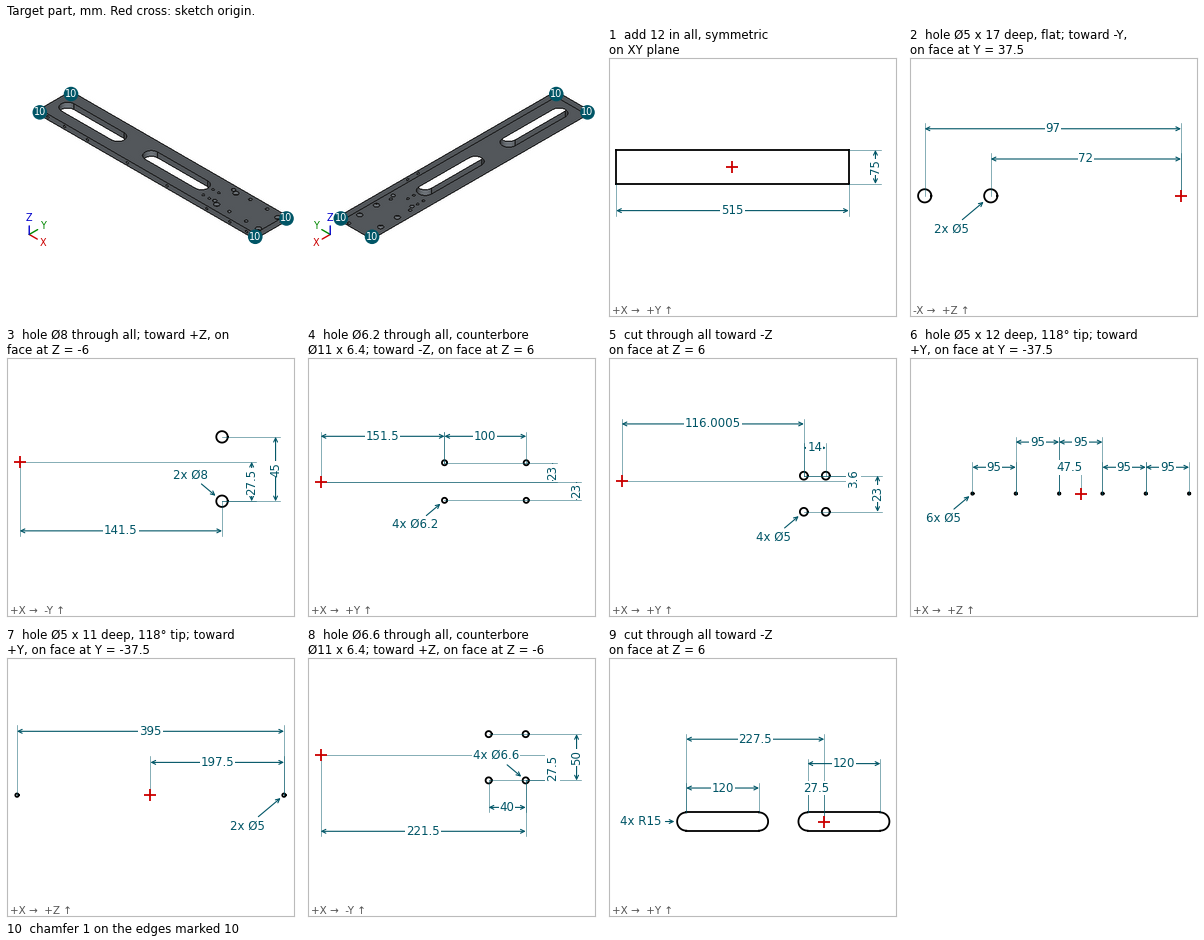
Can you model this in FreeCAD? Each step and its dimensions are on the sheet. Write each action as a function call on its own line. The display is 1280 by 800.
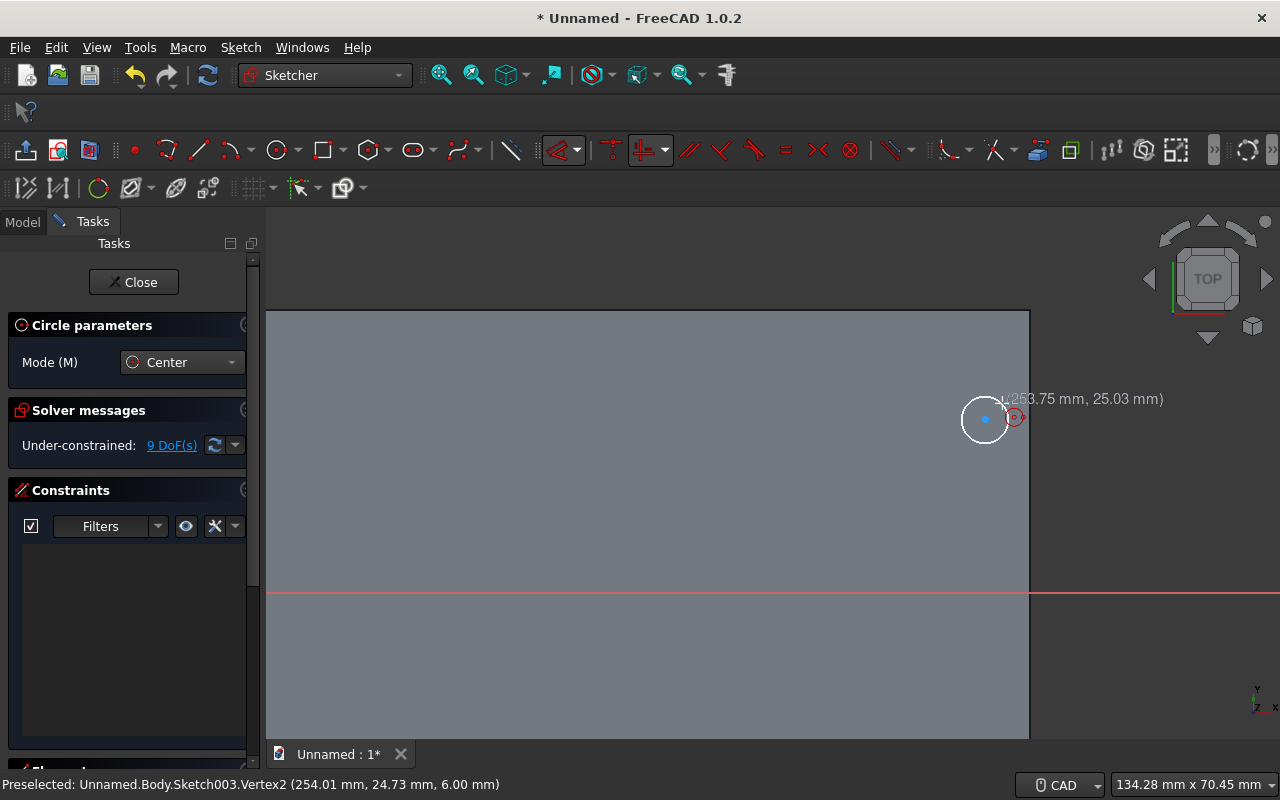
scroll(988, 421, down, 6)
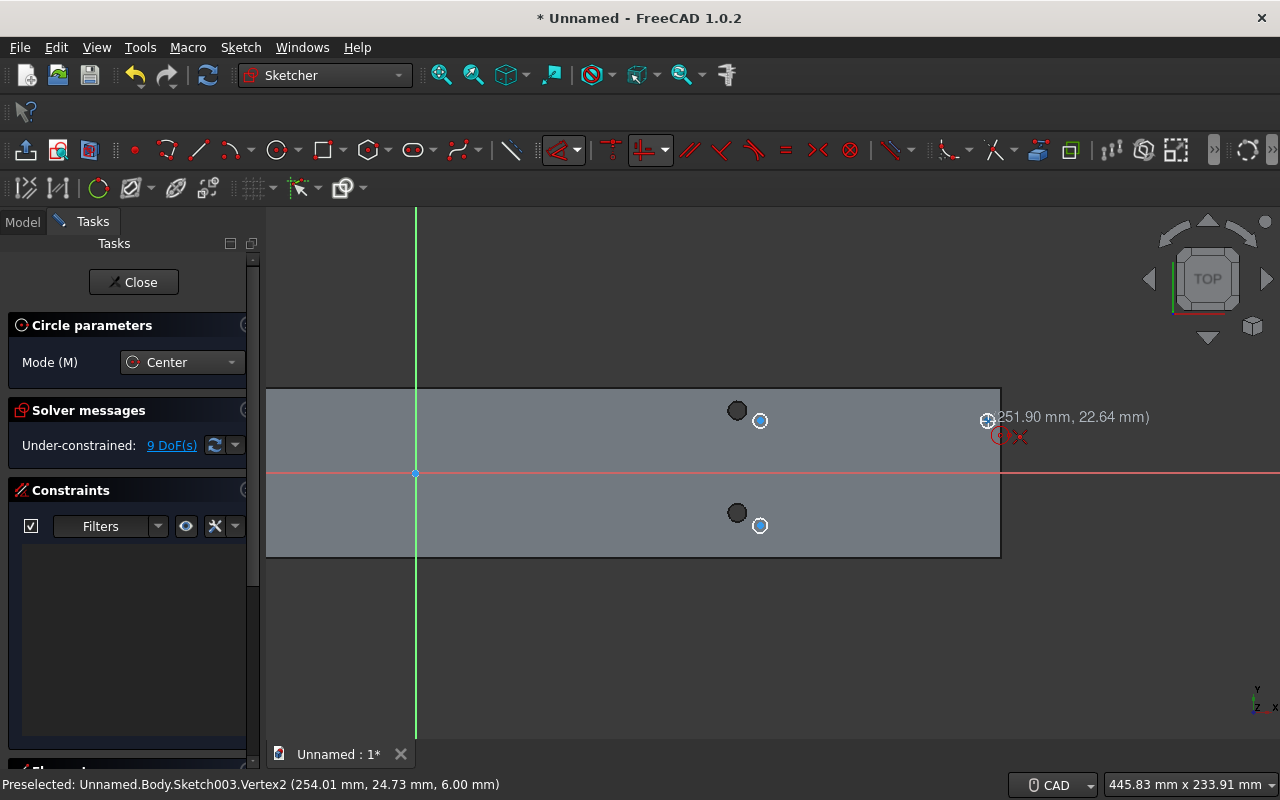
scroll(988, 525, up, 6)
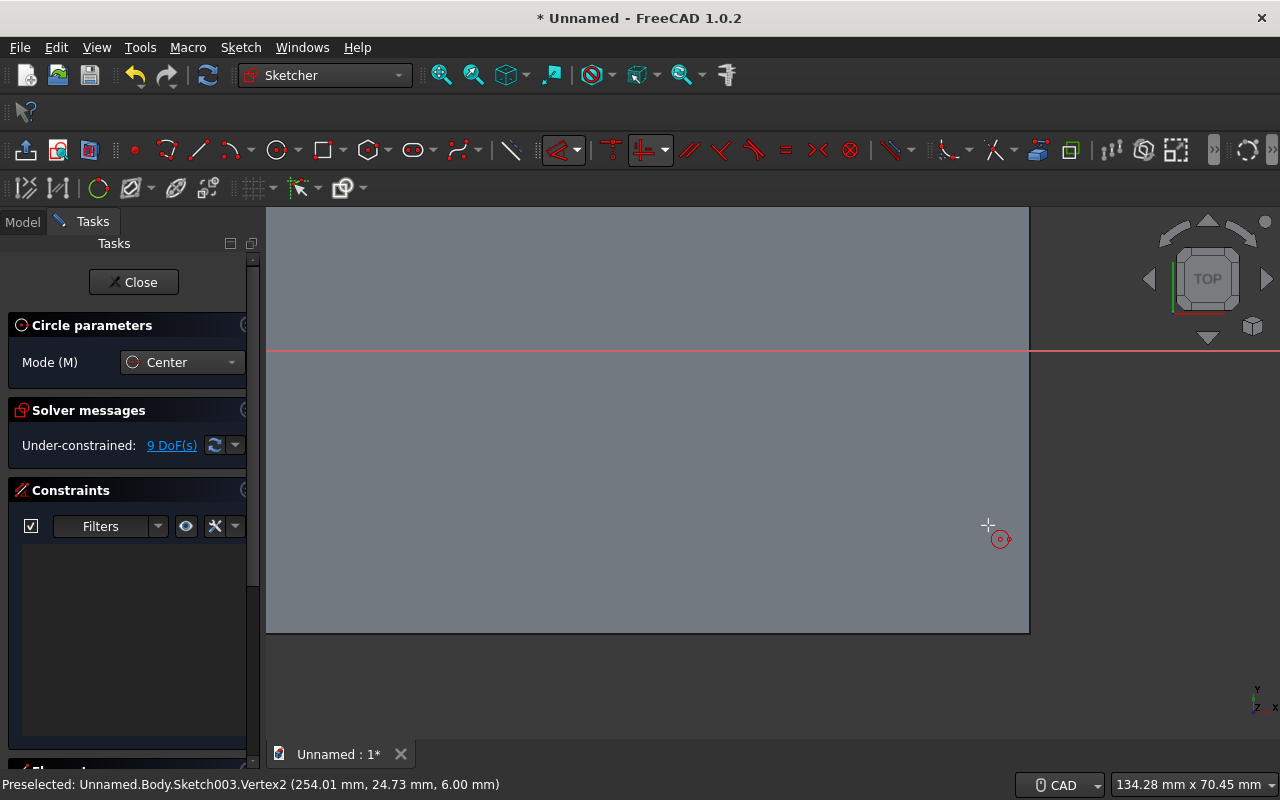
click(985, 525)
click(1002, 508)
key(Escape)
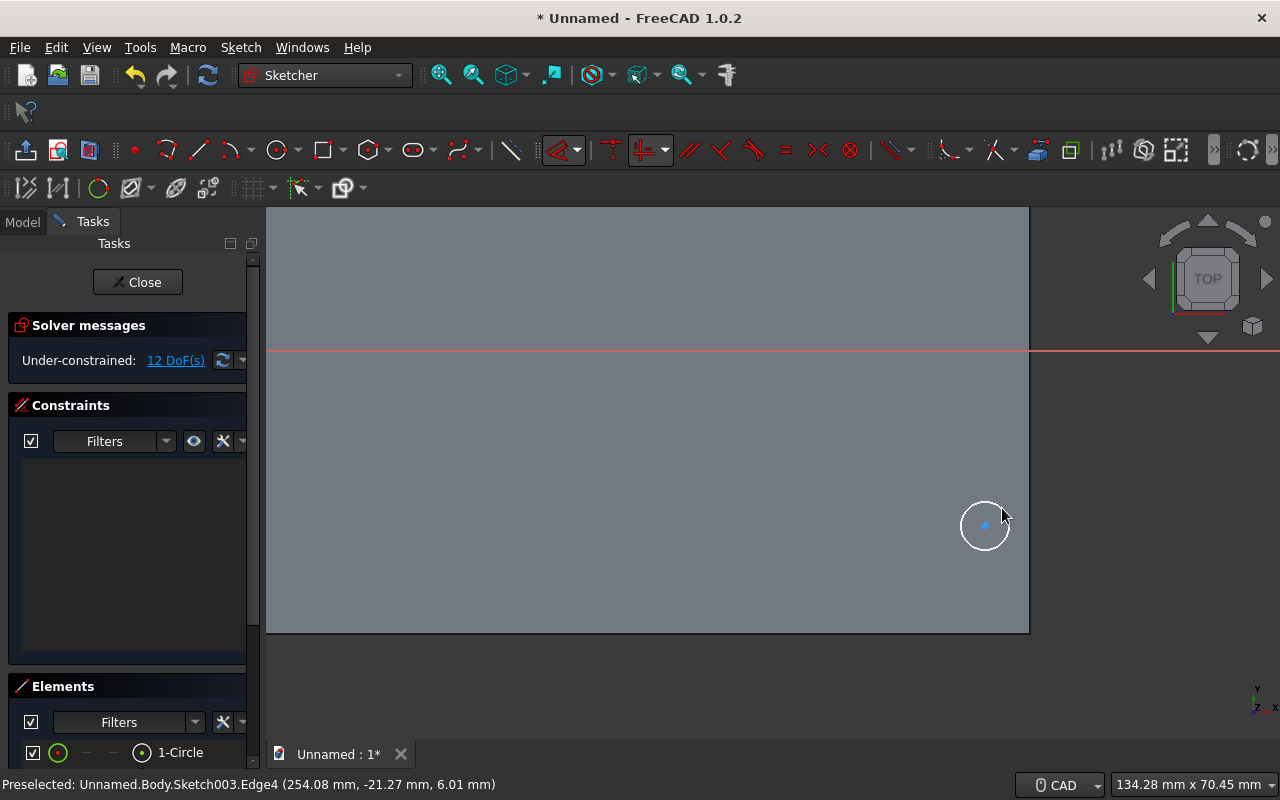
scroll(988, 525, down, 6)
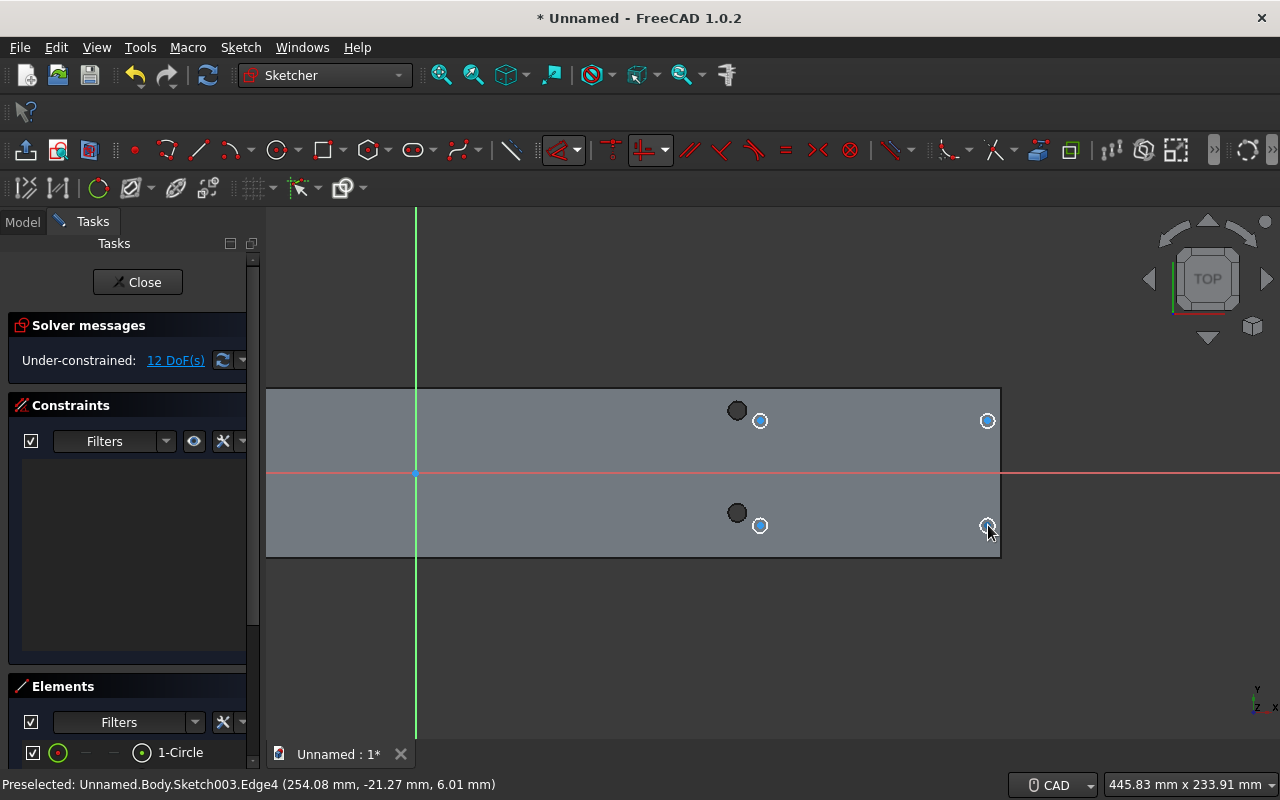
scroll(765, 416, up, 4)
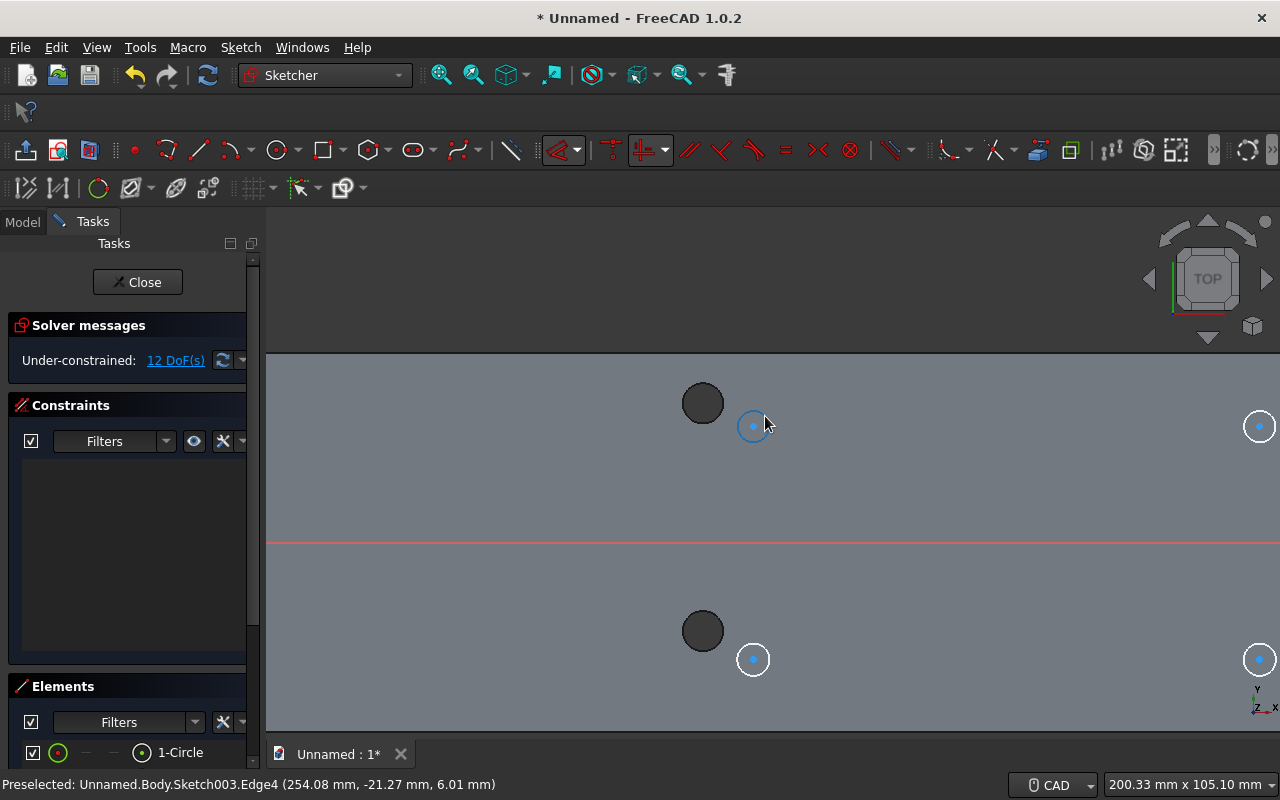
click(765, 416)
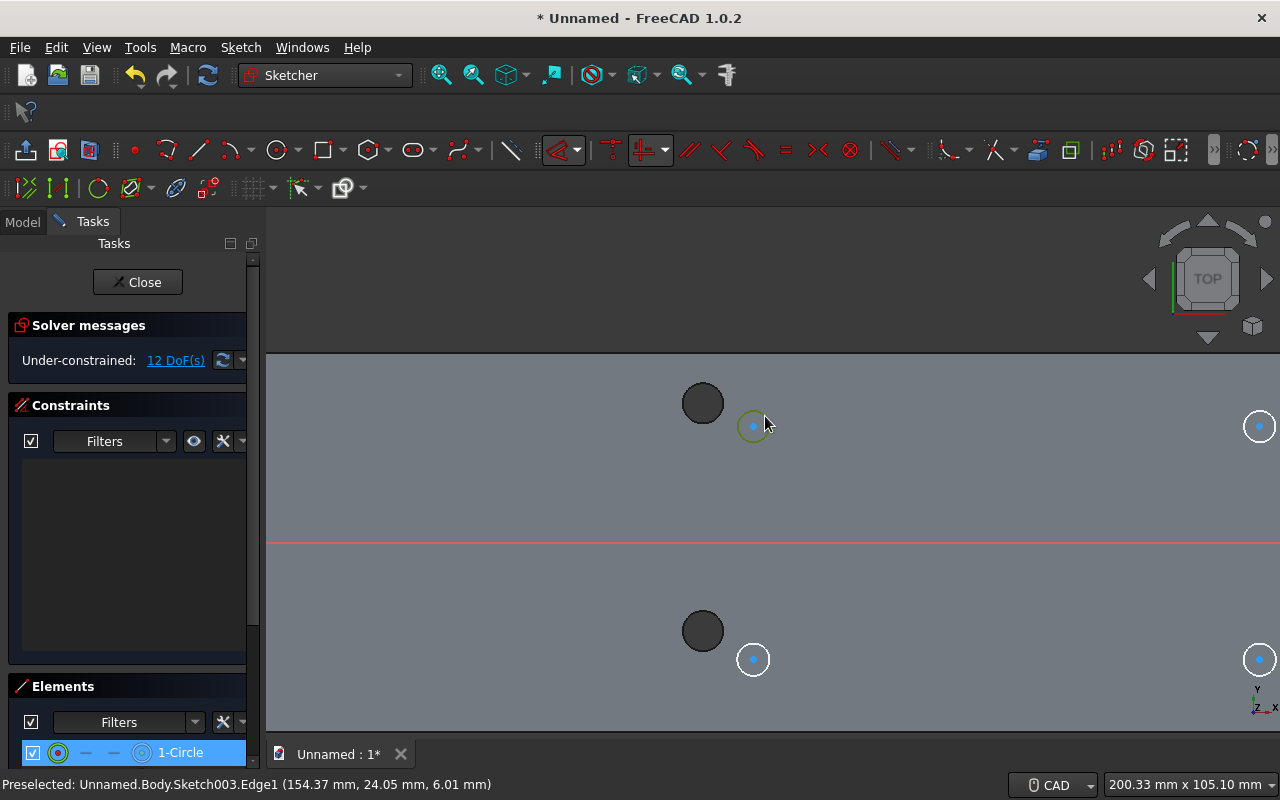
click(765, 648)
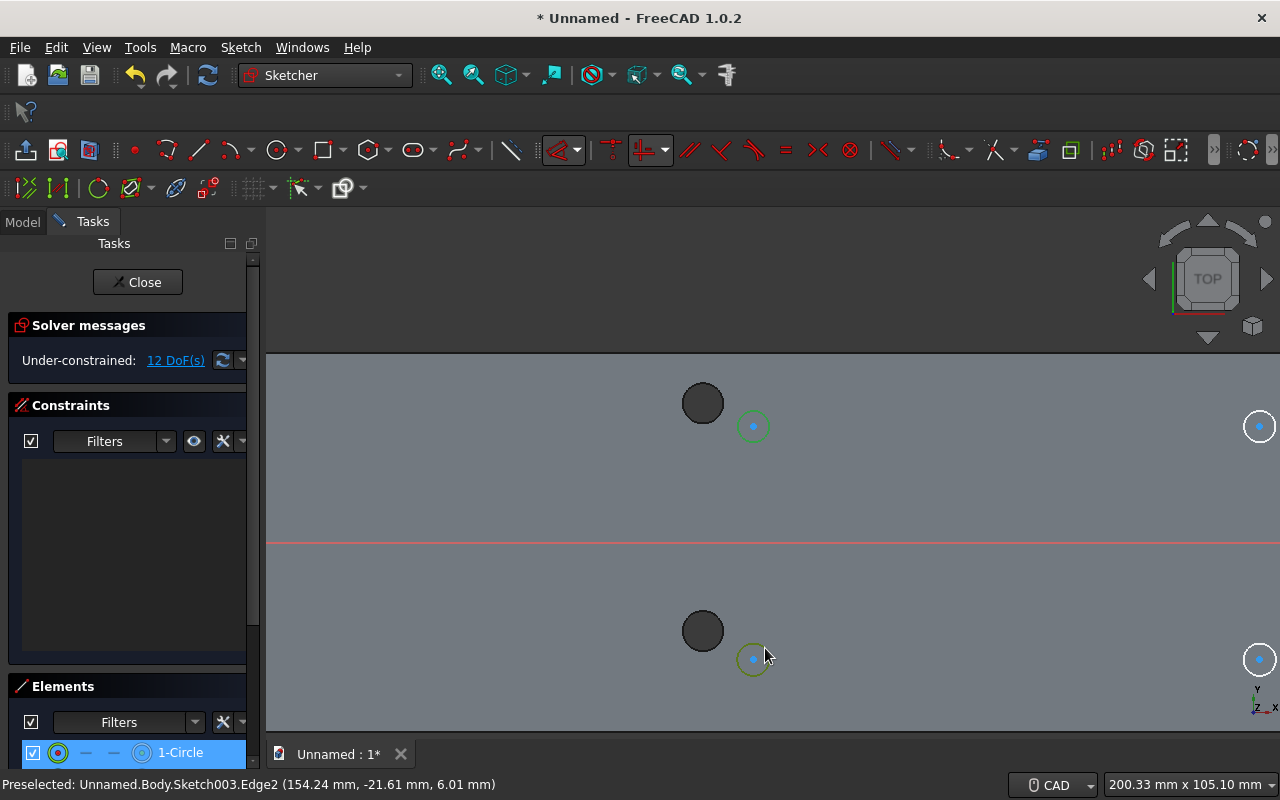
scroll(764, 416, down, 4)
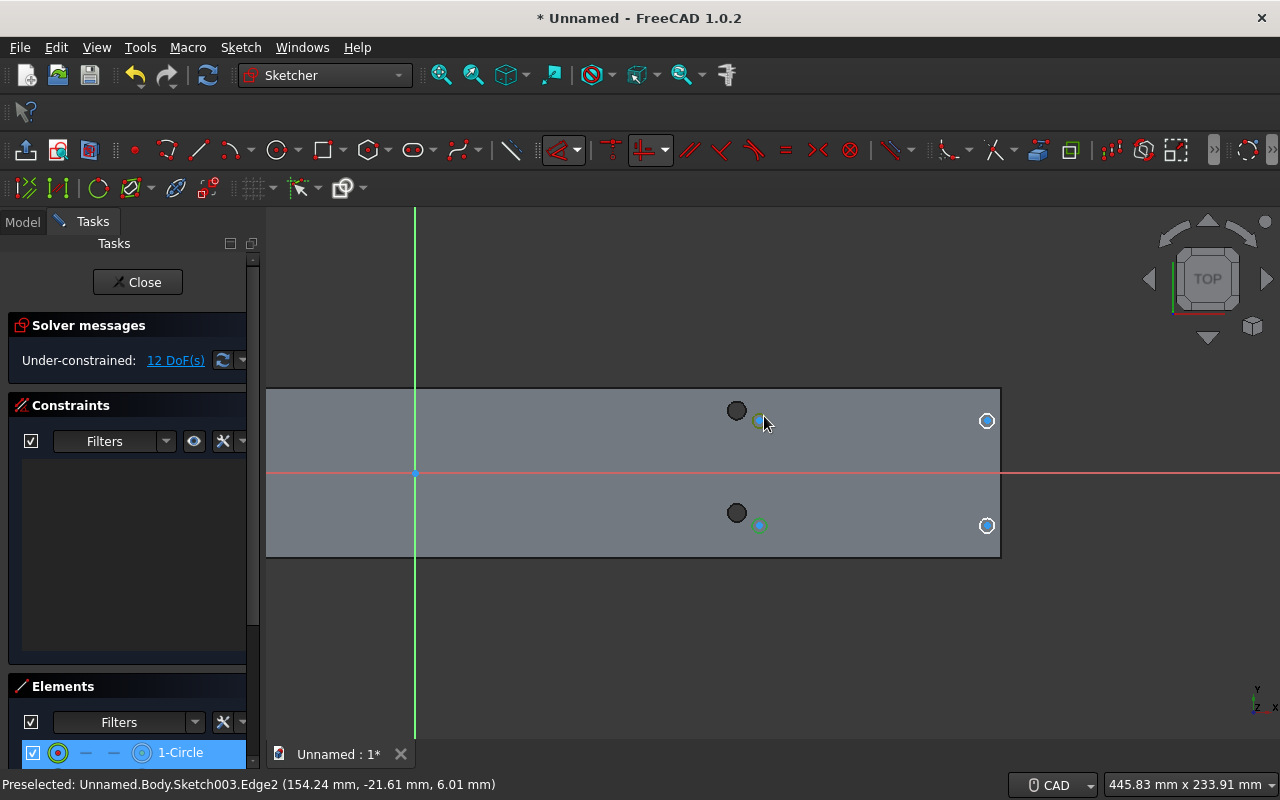
scroll(992, 416, up, 4)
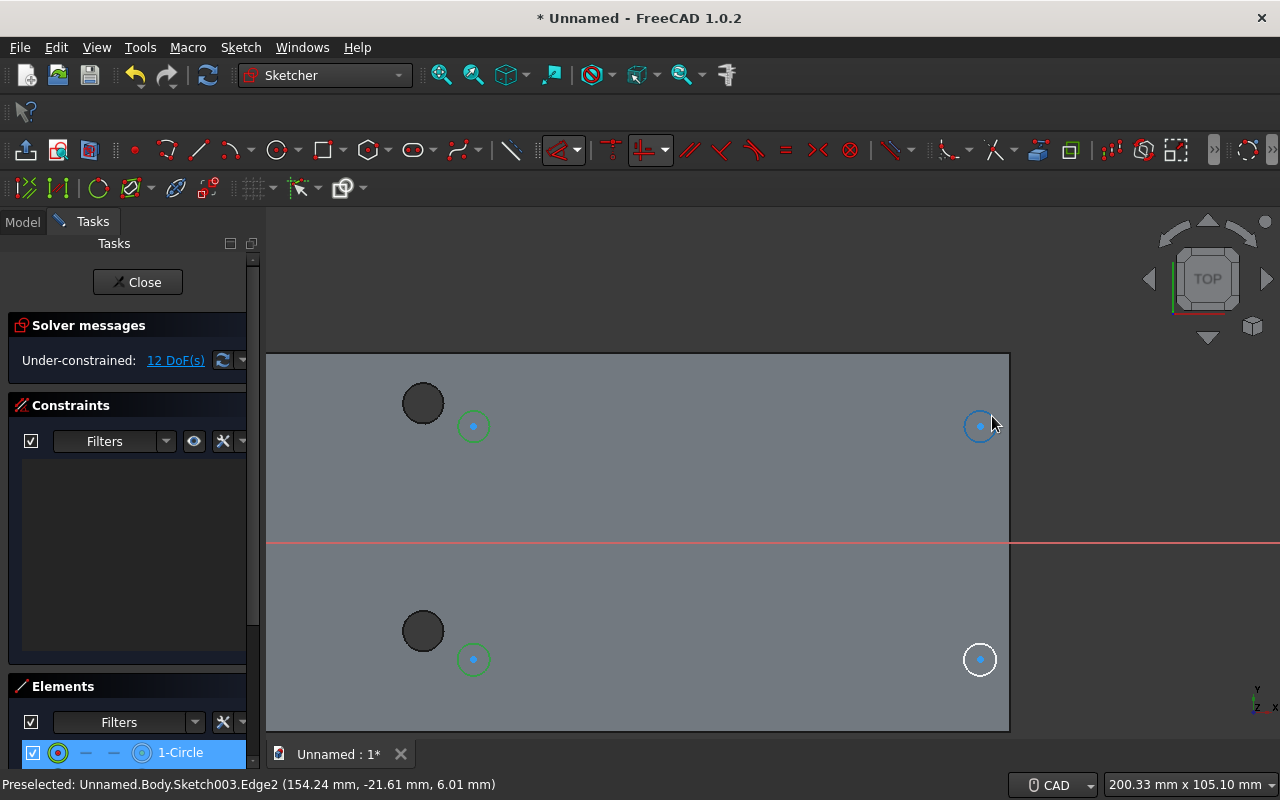
click(991, 416)